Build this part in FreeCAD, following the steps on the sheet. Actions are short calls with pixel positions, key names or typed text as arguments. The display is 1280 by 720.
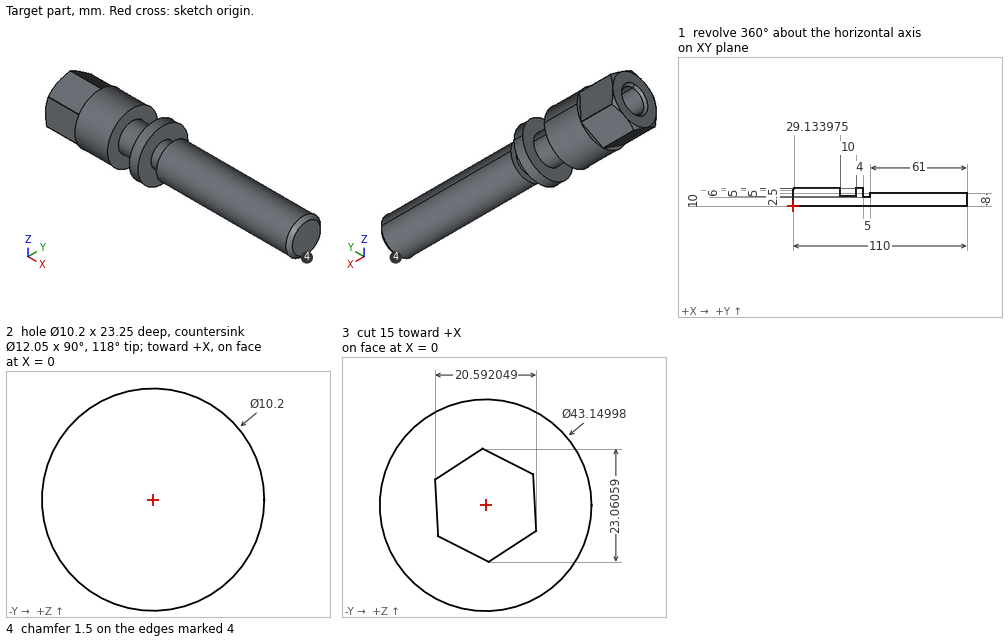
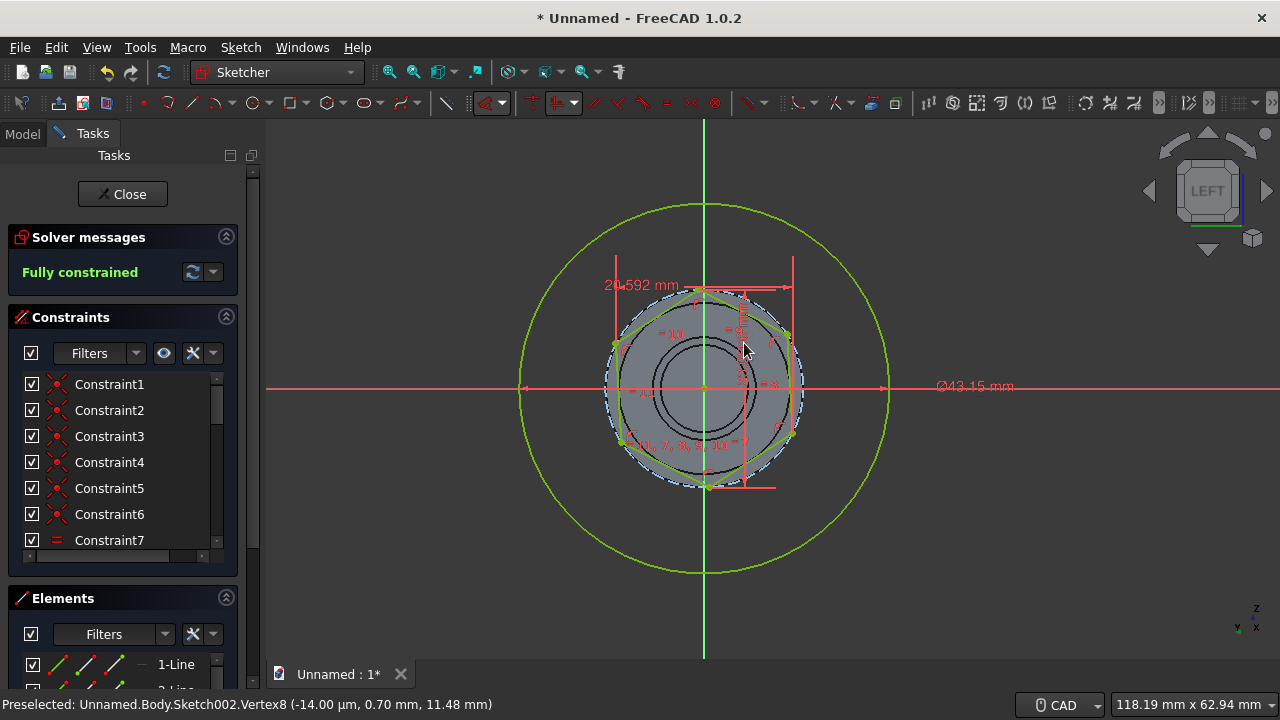
click(123, 194)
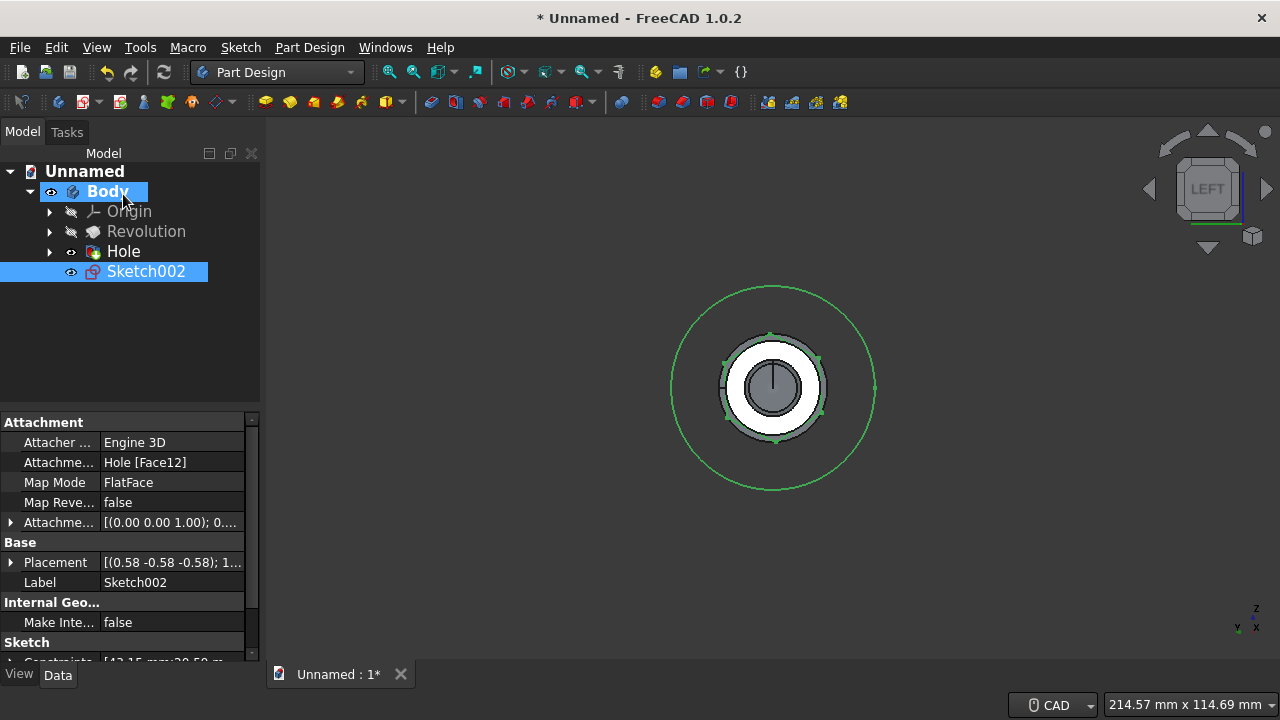
click(432, 102)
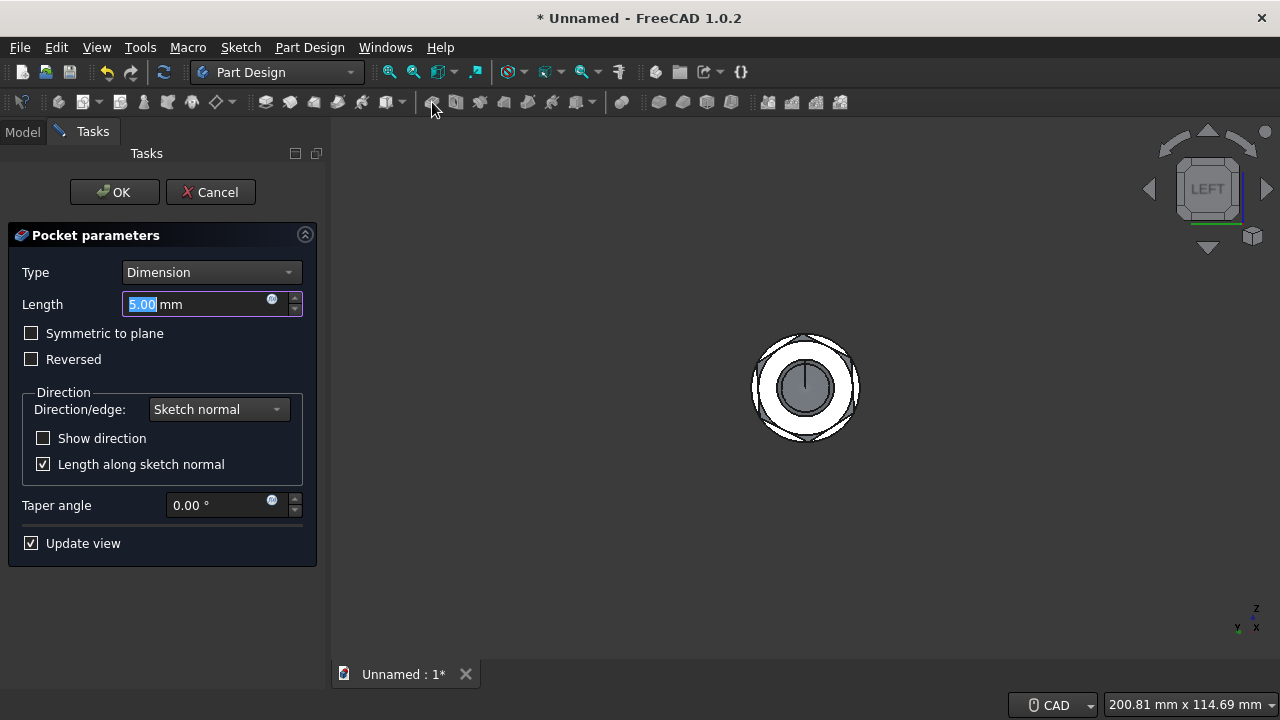
text(15)
key(Tab)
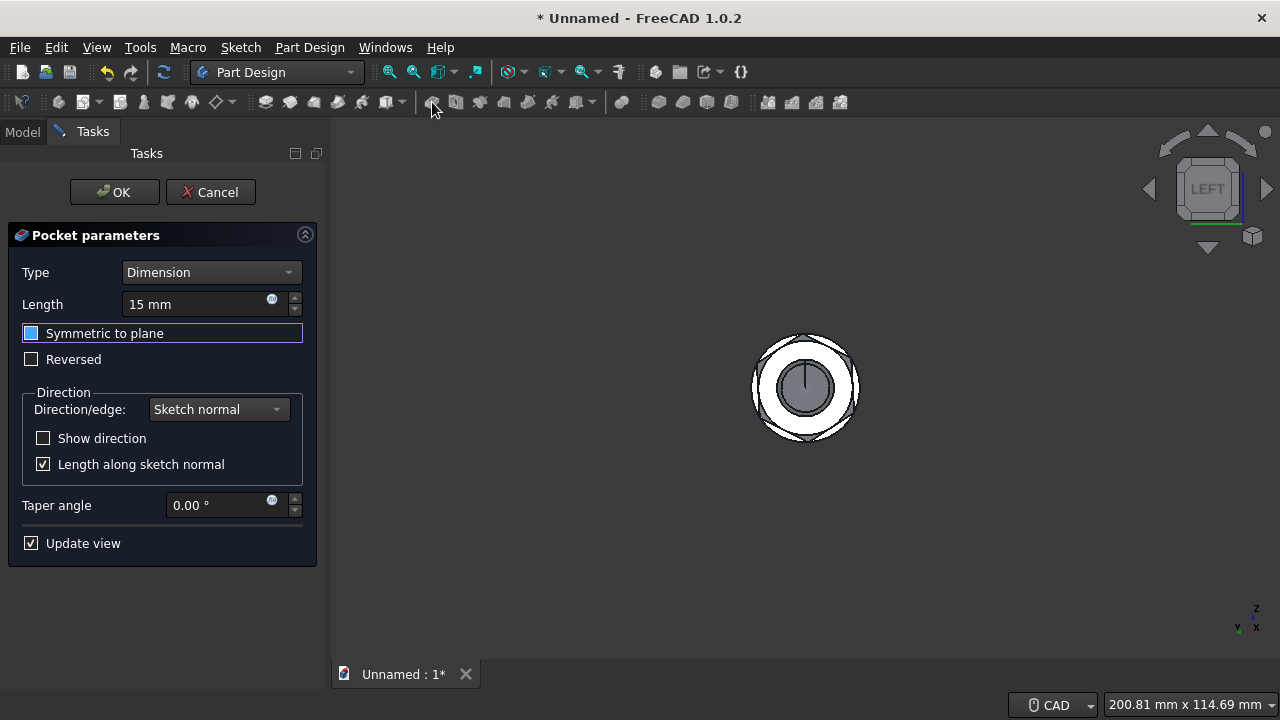
click(115, 192)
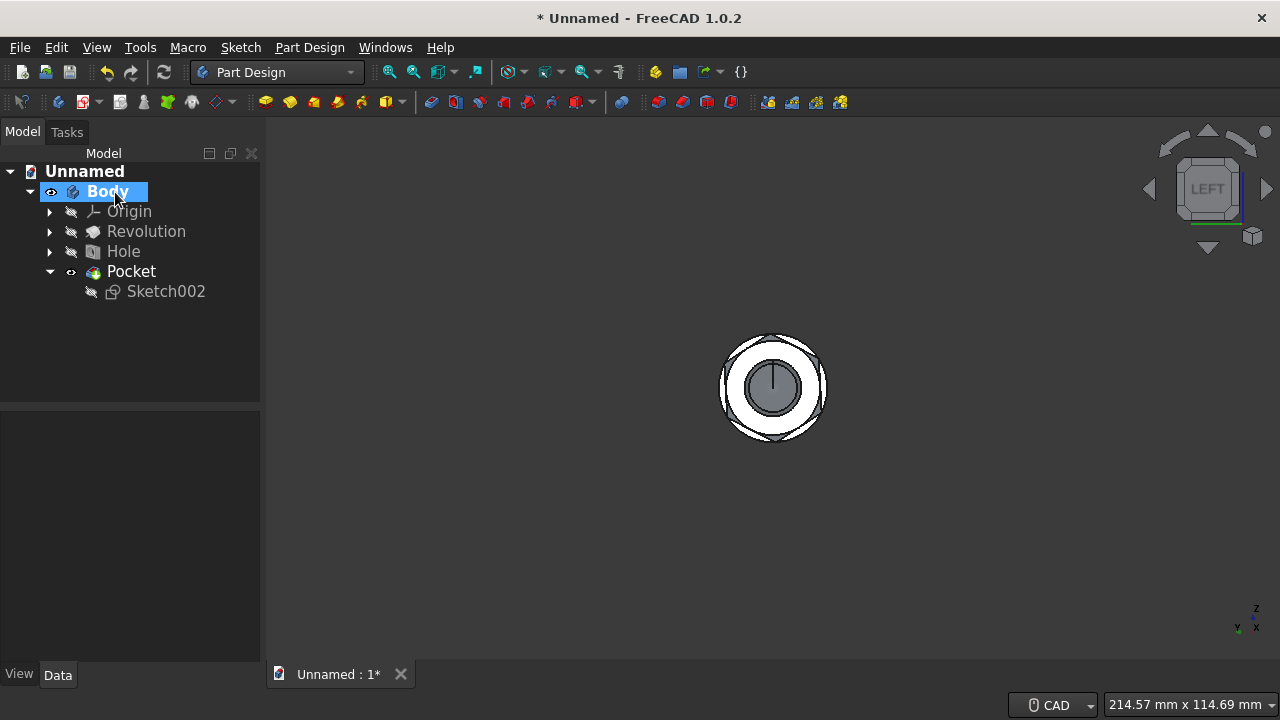
click(390, 72)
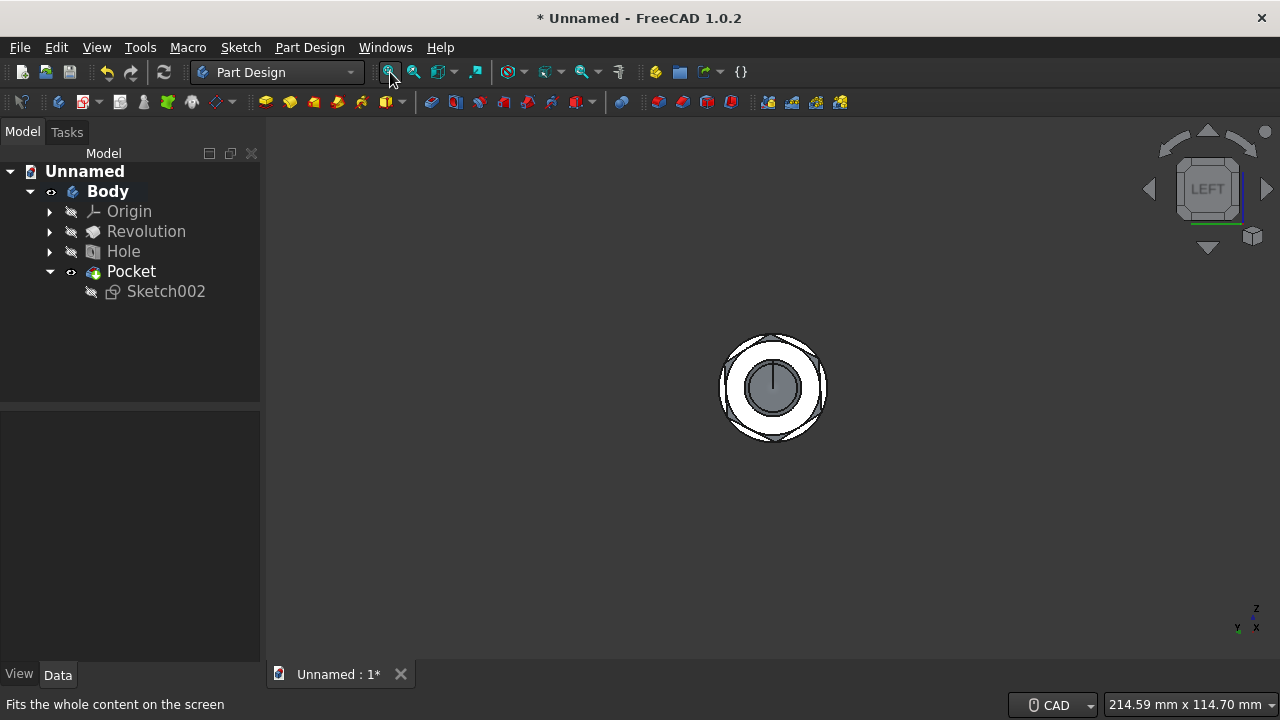
key(0)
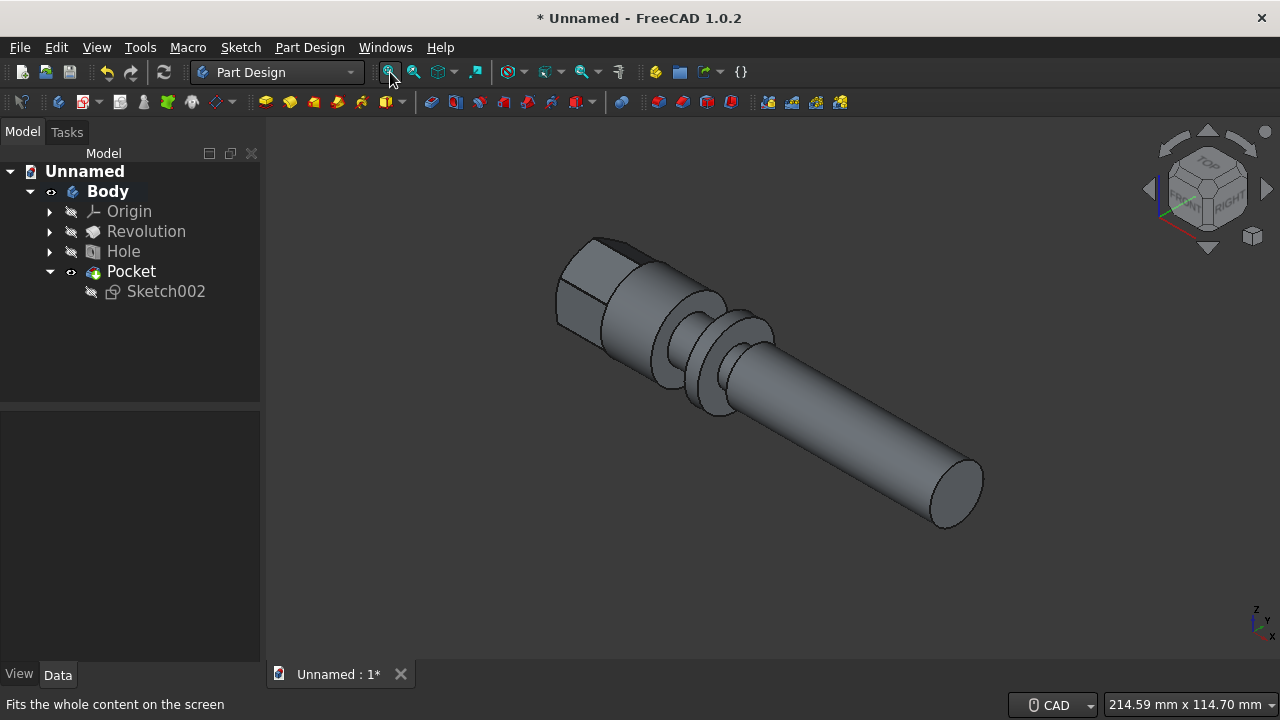
click(930, 509)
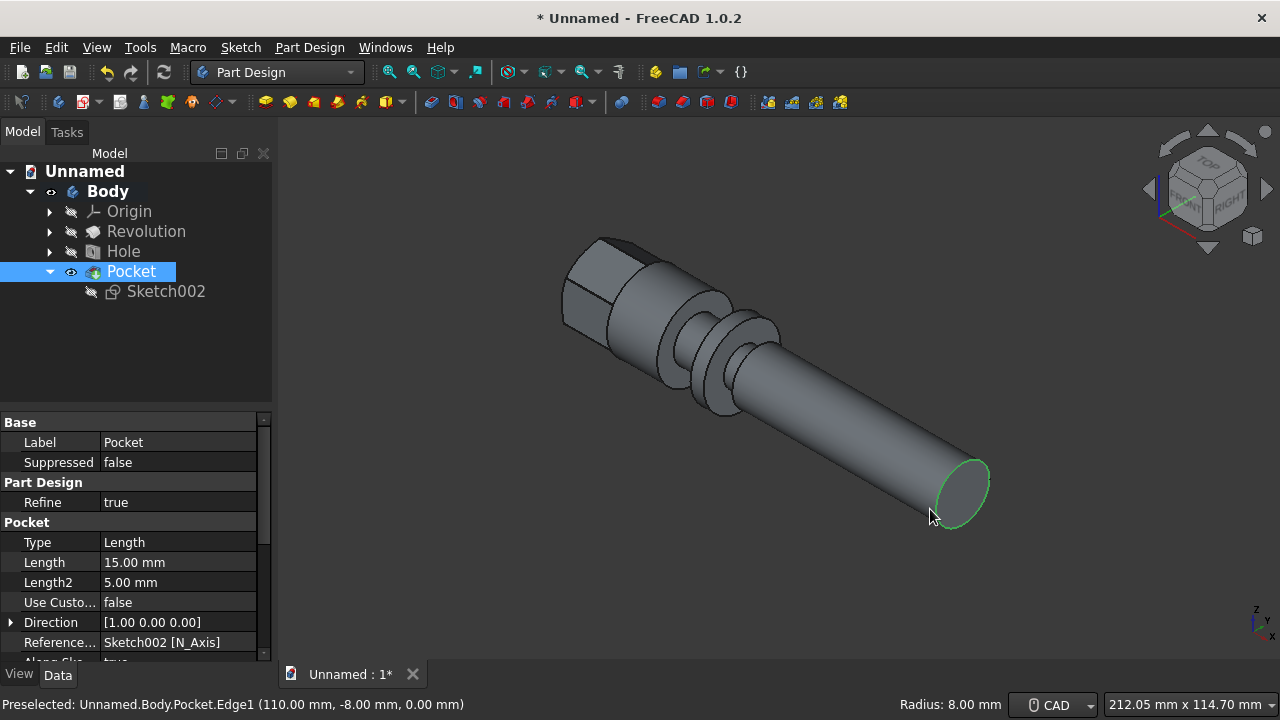
click(684, 102)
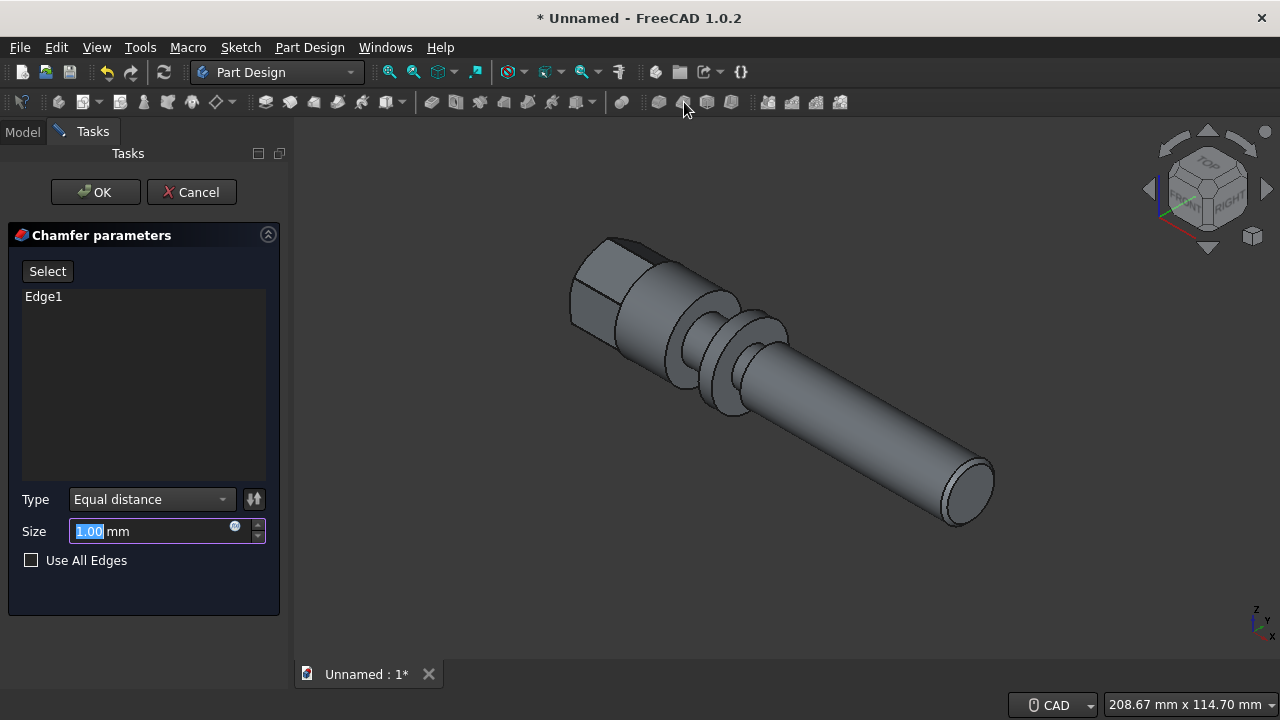
text(1.5)
key(Tab)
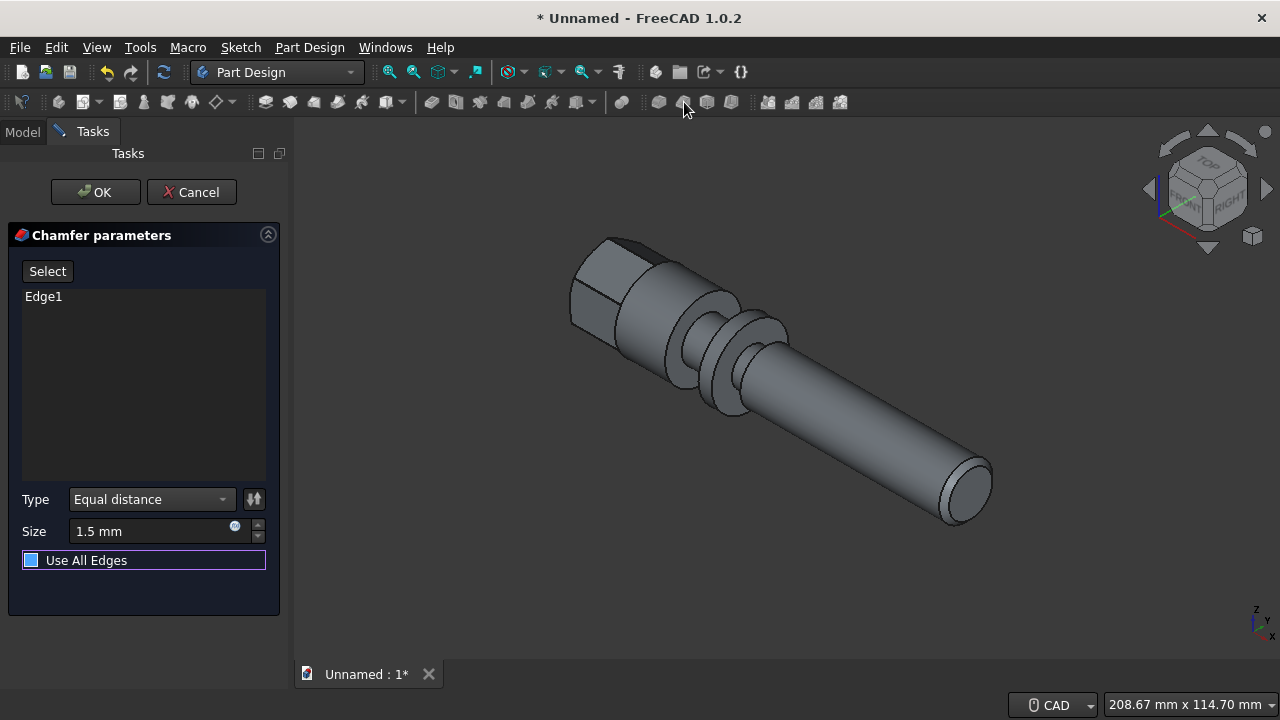
click(96, 192)